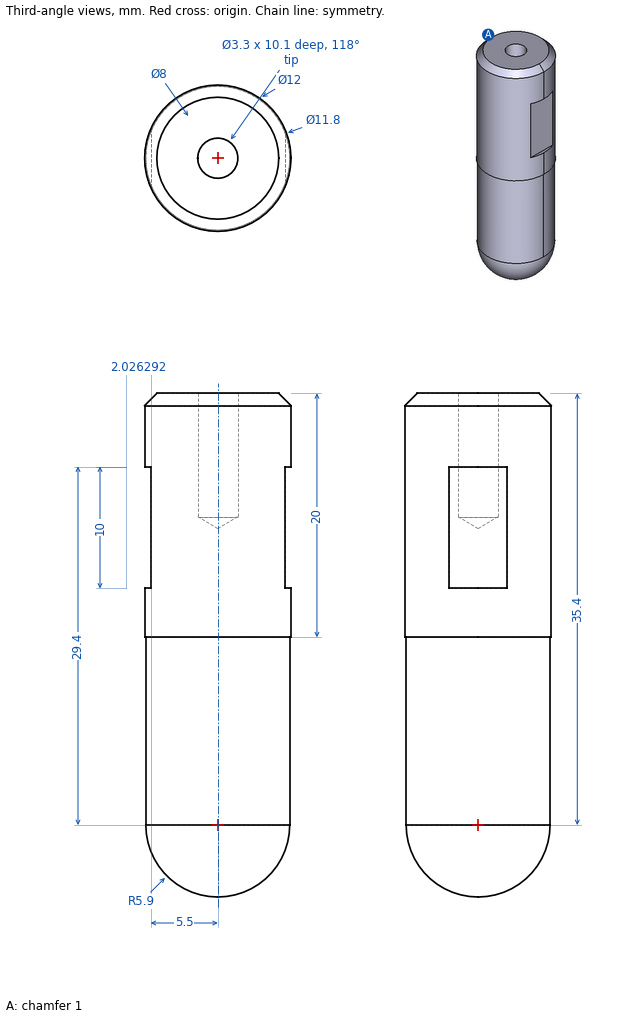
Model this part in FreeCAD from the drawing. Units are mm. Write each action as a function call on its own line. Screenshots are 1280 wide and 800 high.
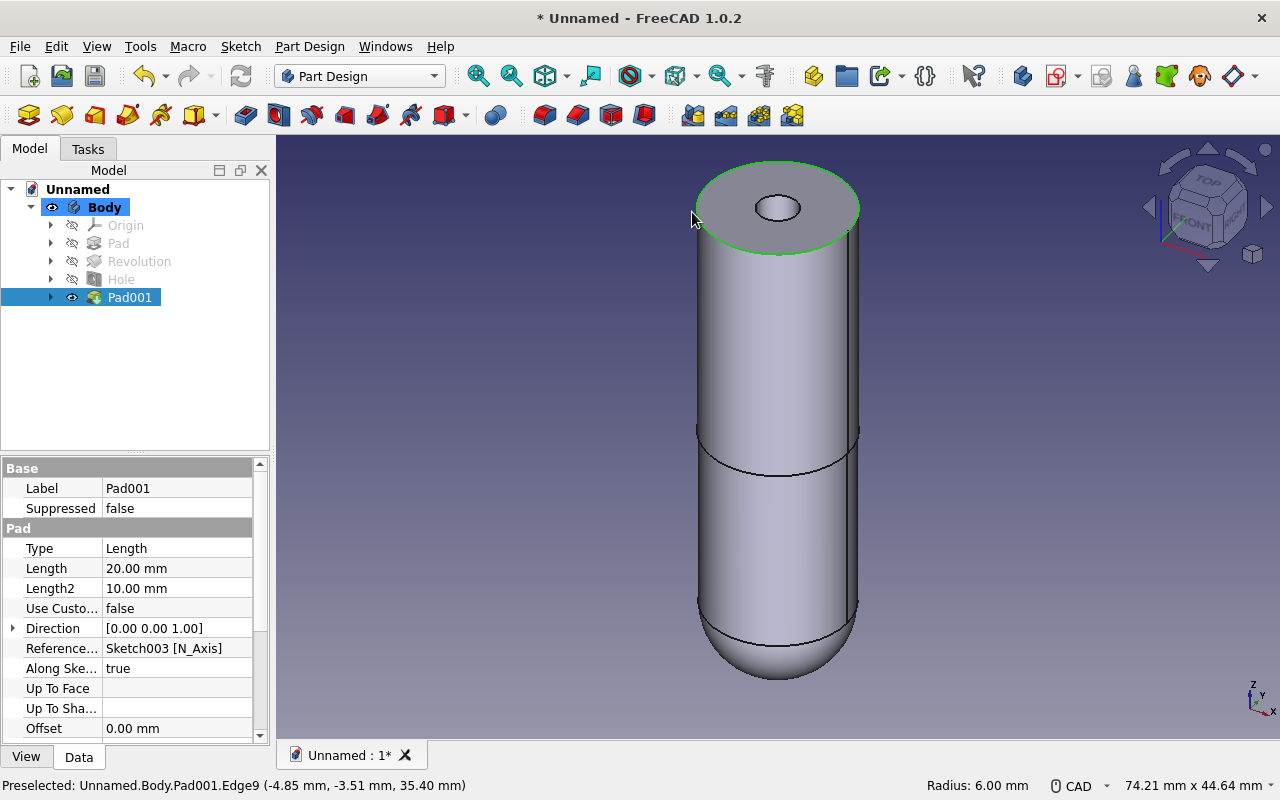
click(578, 116)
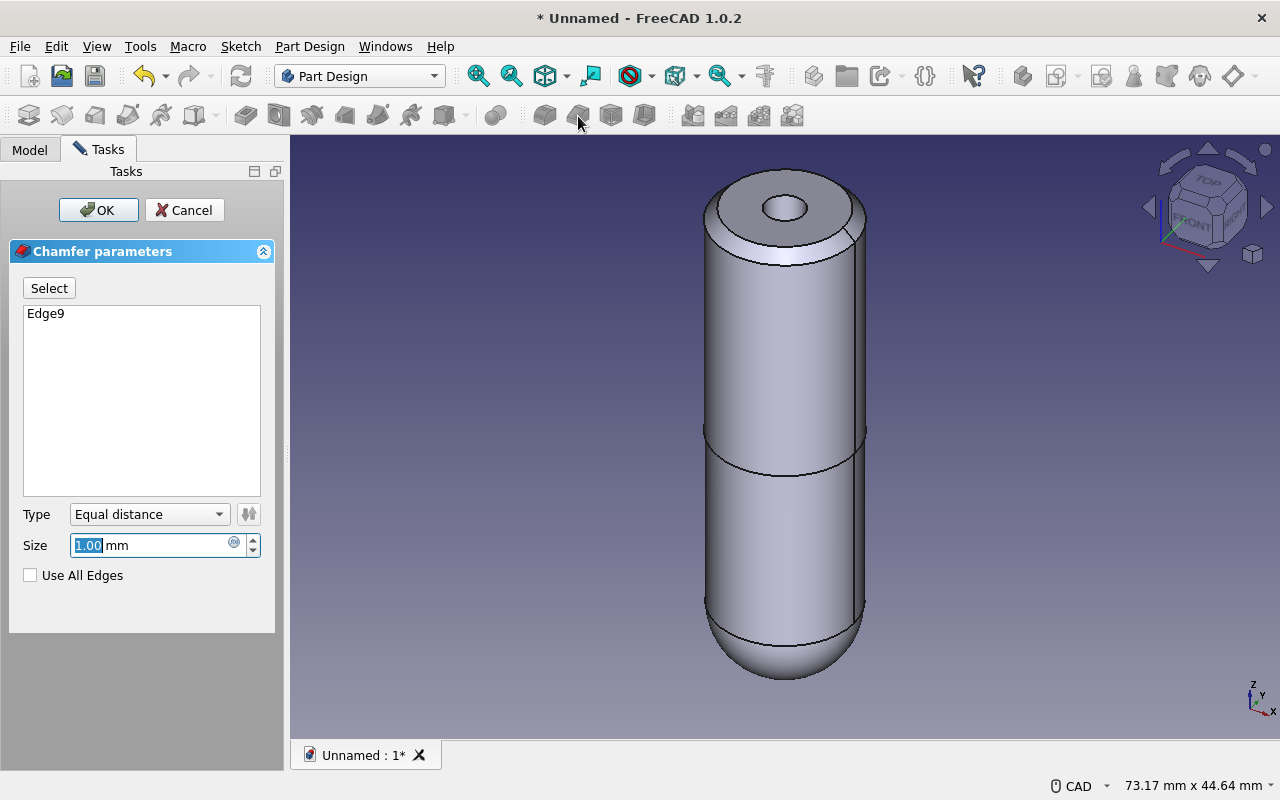
text(1)
key(Tab)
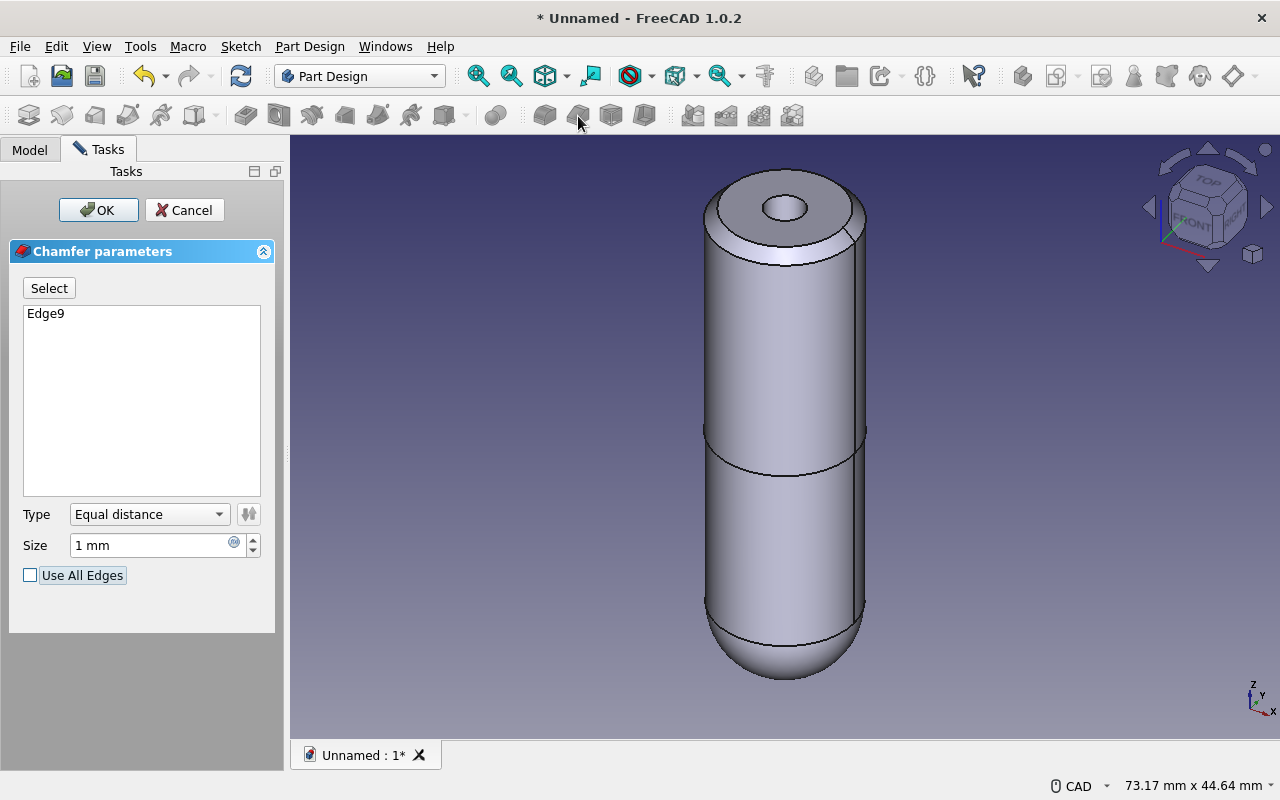
click(99, 210)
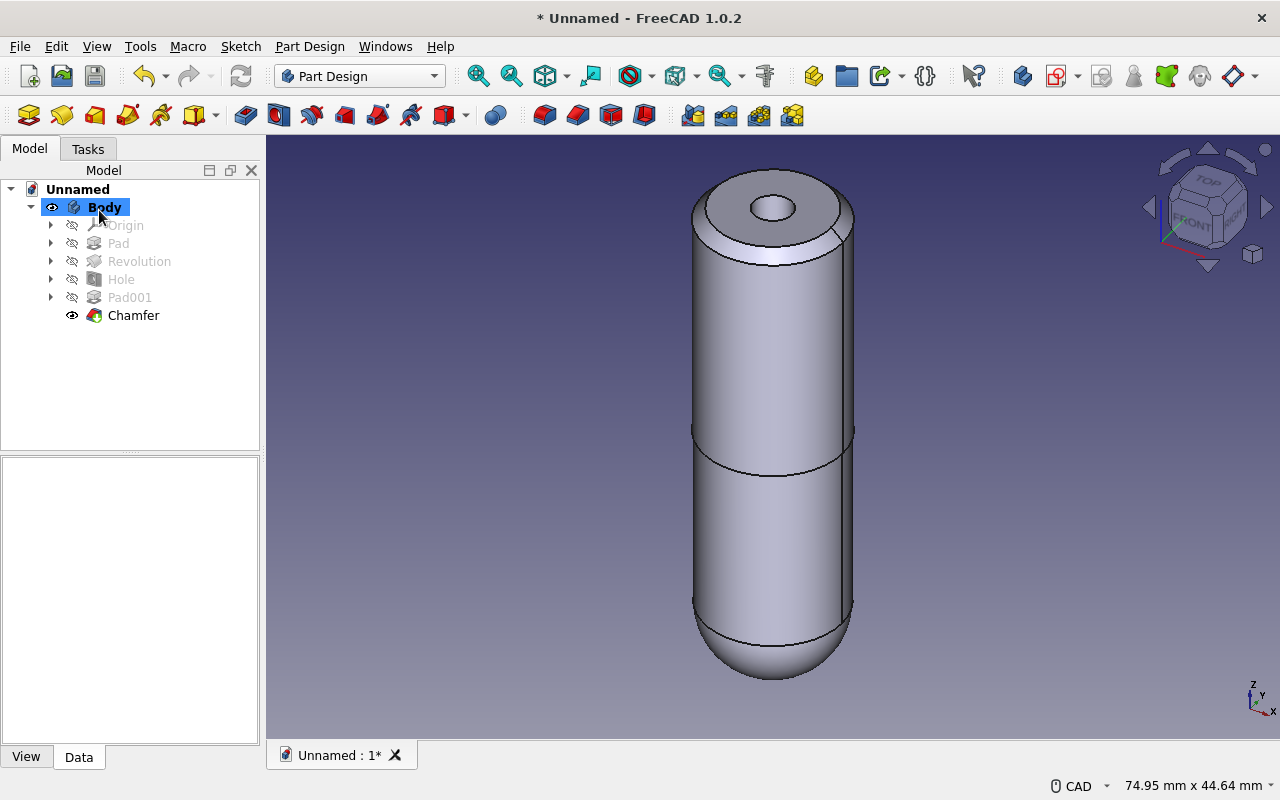
click(1056, 76)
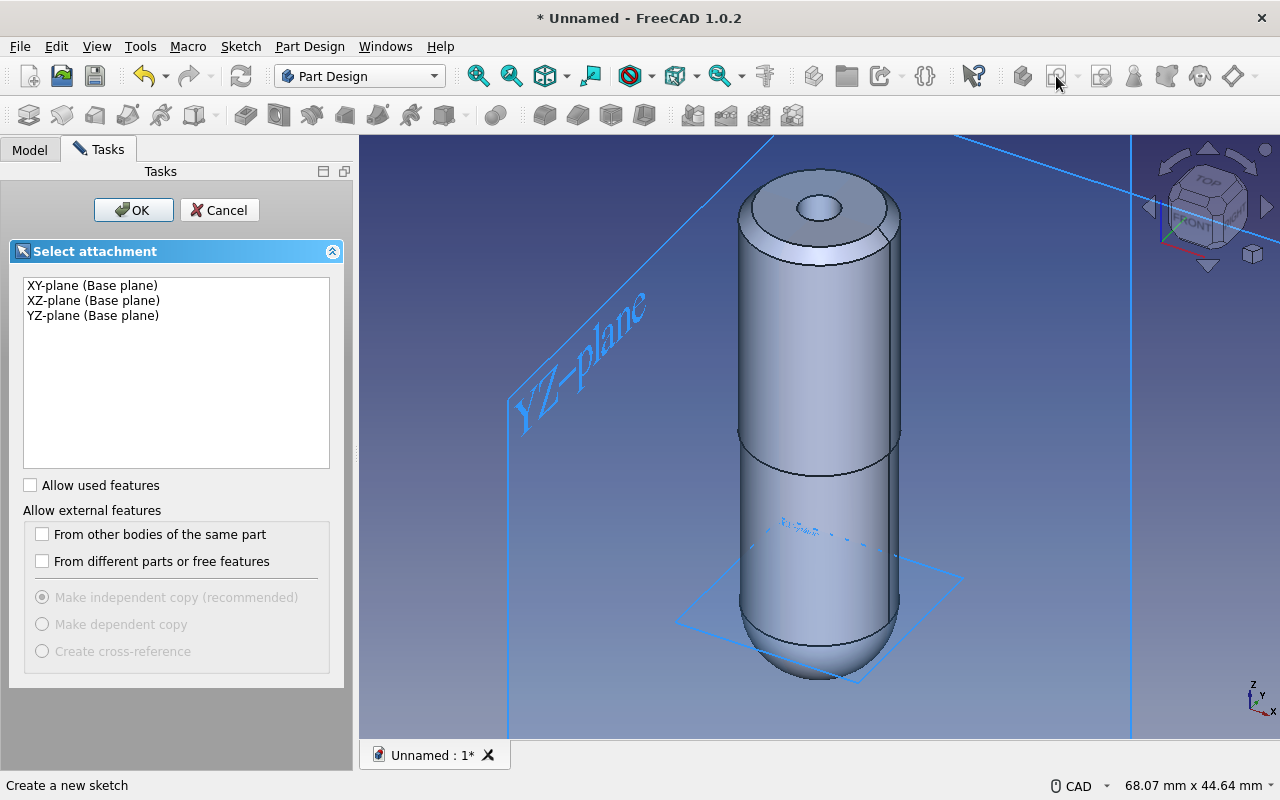
click(84, 300)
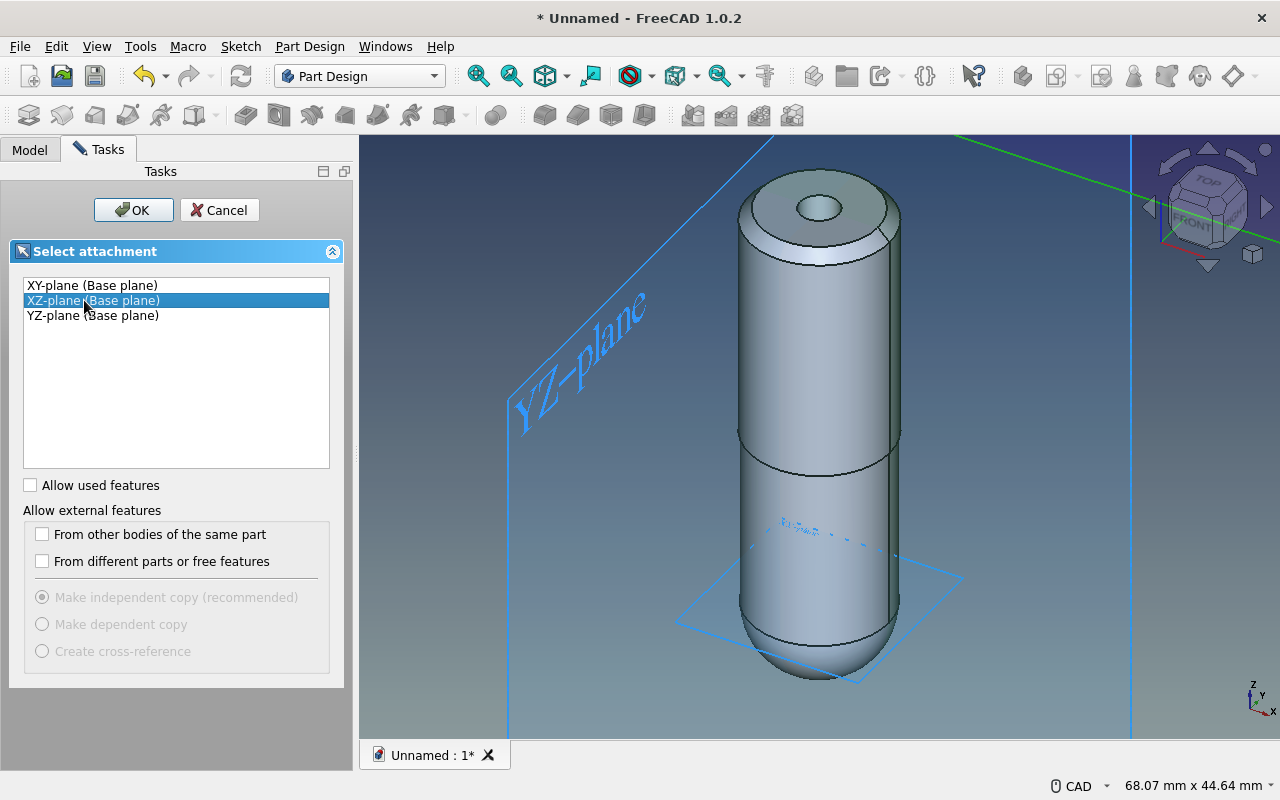
click(134, 210)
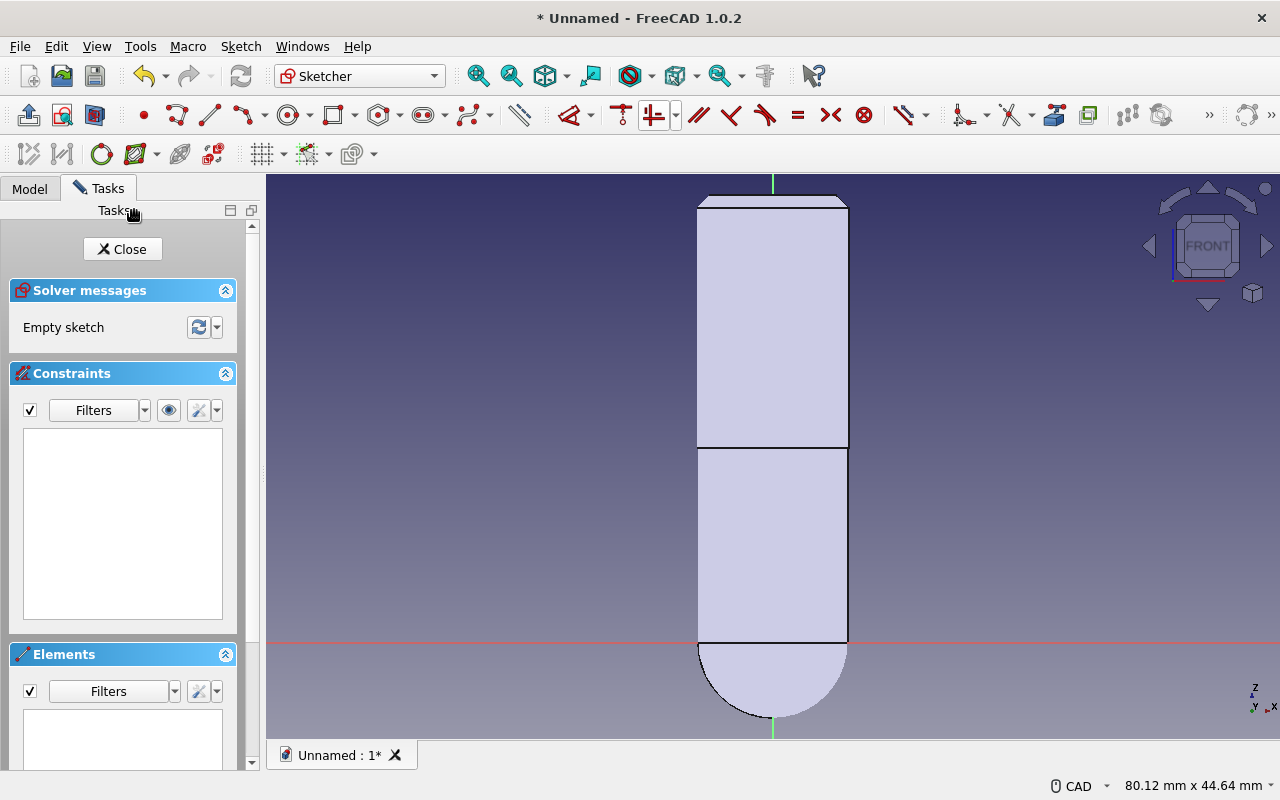
click(95, 116)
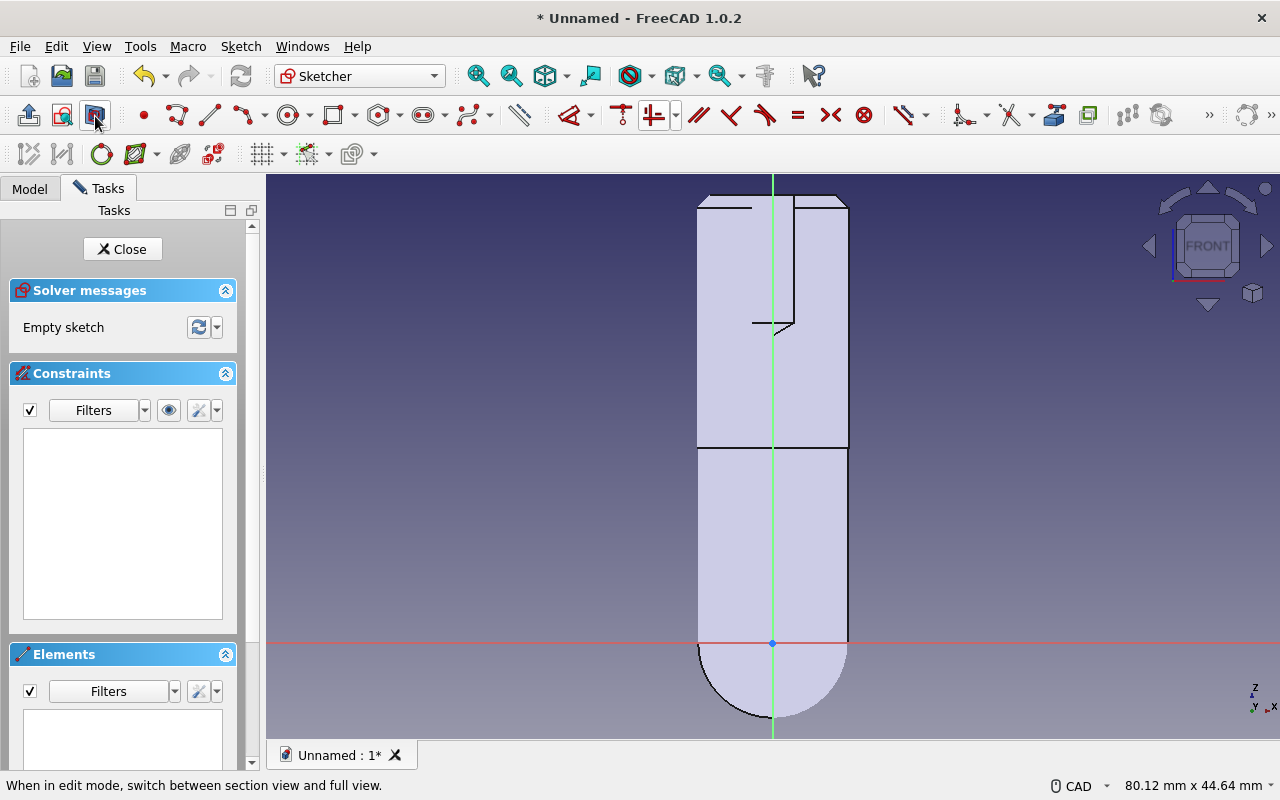
click(332, 116)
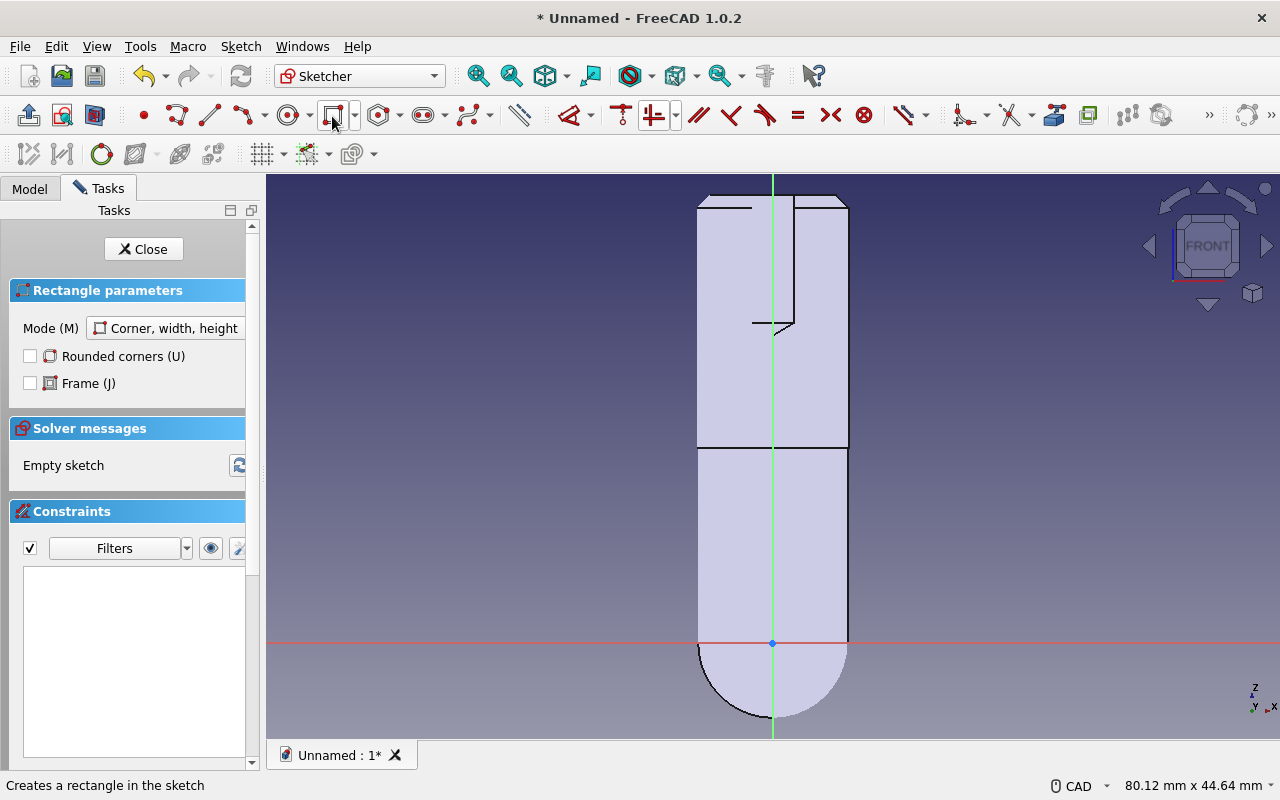
click(678, 271)
click(703, 398)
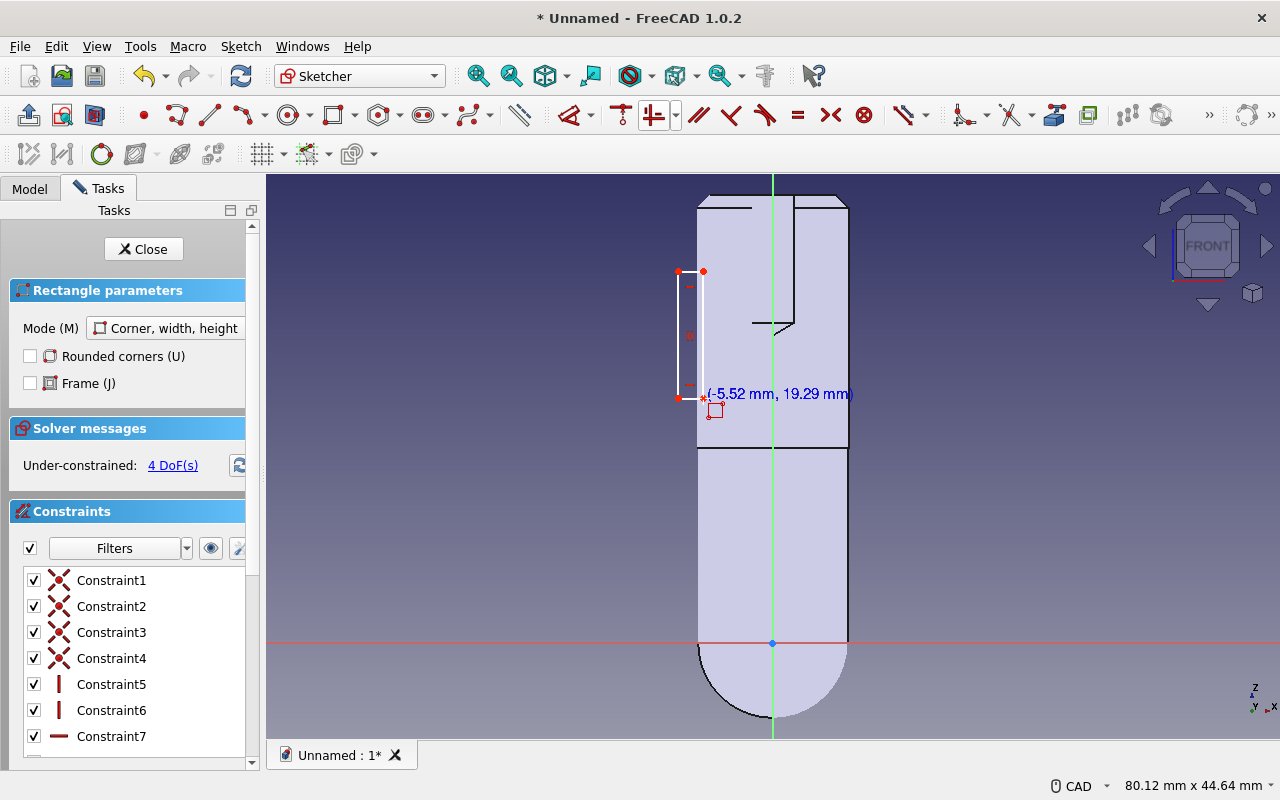
click(842, 271)
click(868, 398)
key(Escape)